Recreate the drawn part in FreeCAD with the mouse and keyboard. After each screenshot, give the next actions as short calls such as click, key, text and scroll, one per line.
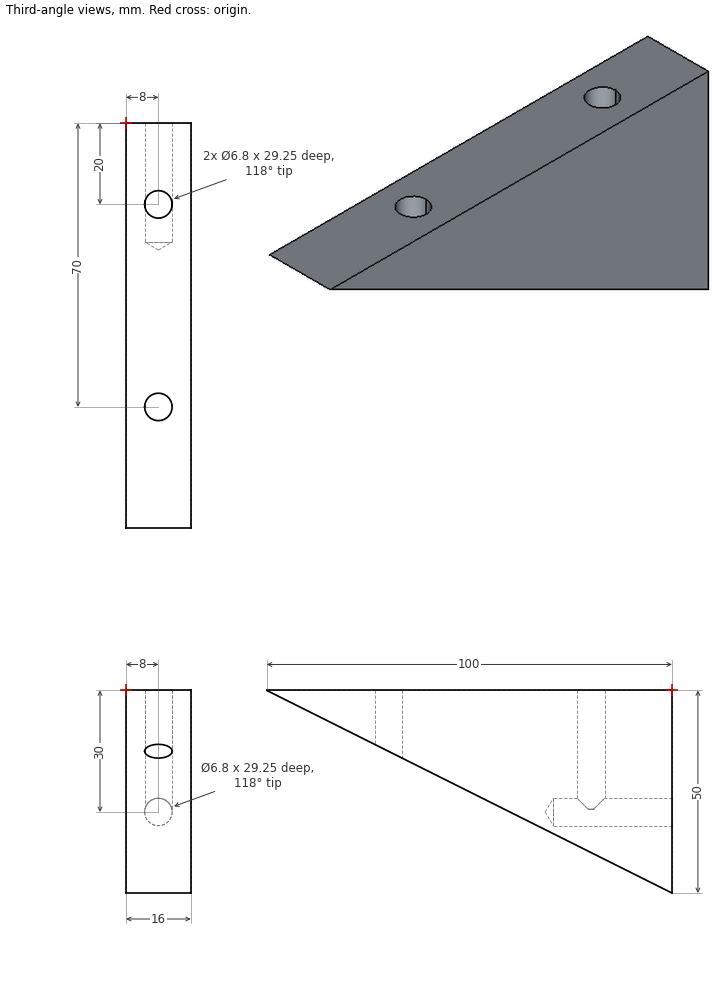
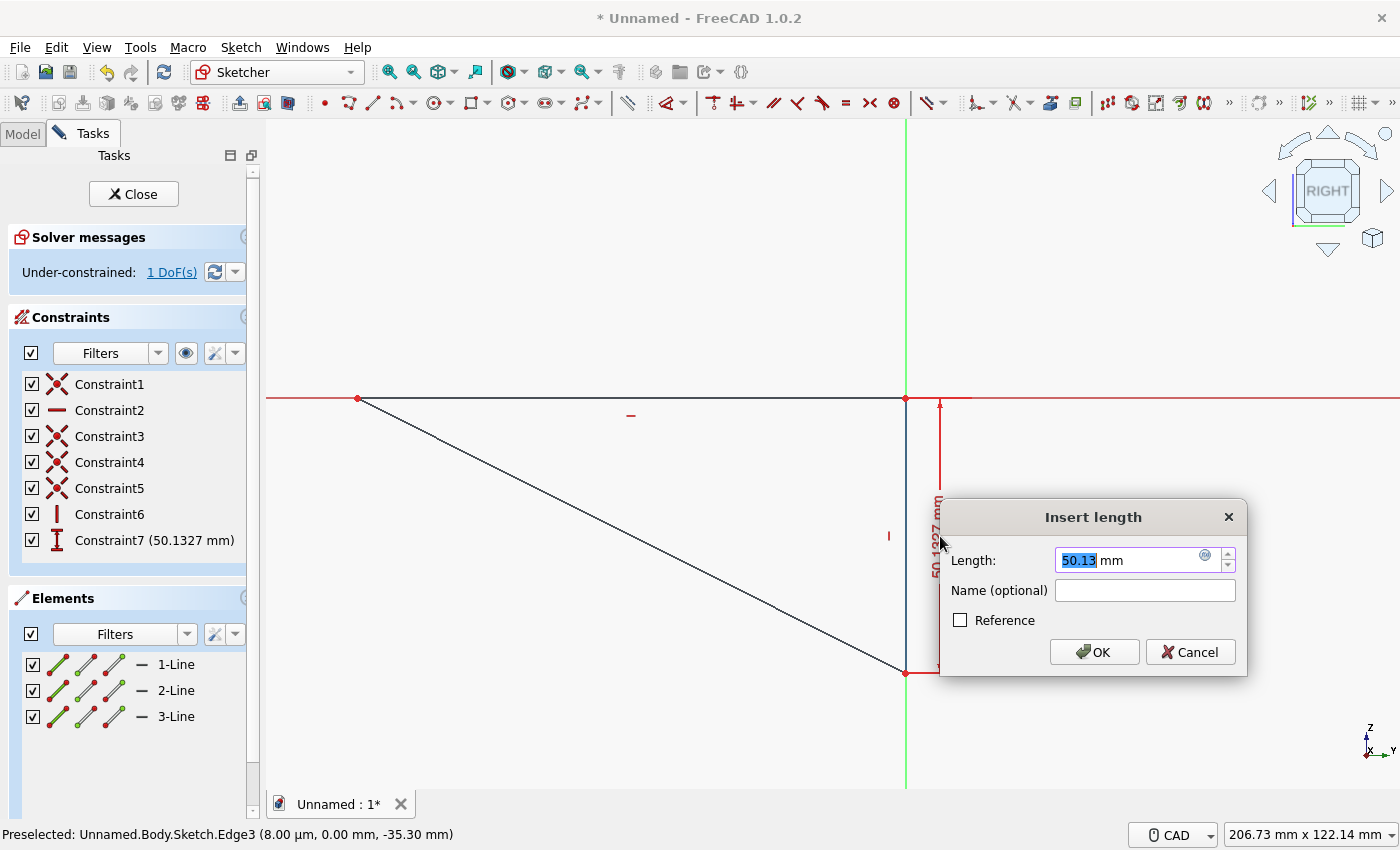
text(50)
key(Return)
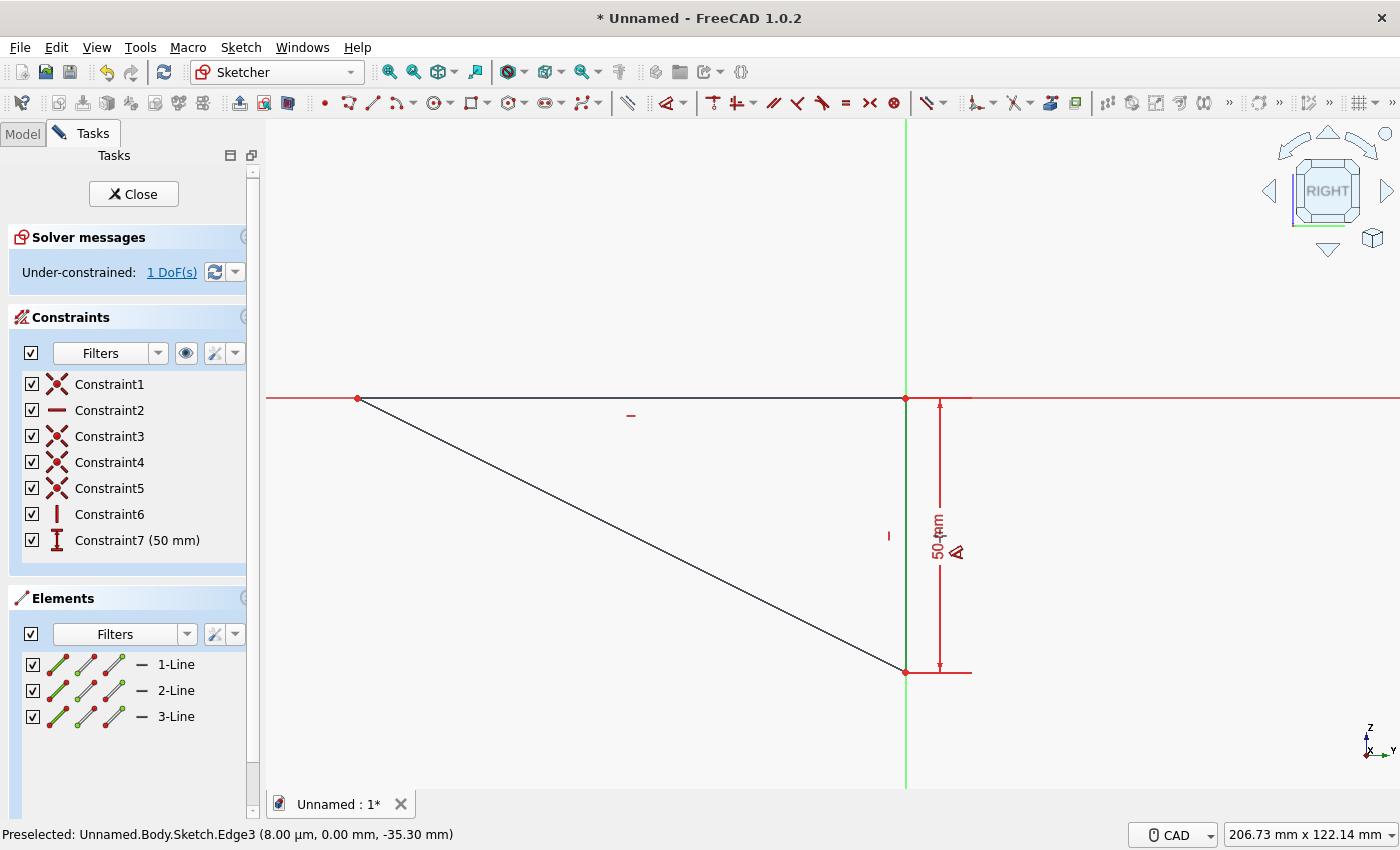
click(741, 398)
click(632, 364)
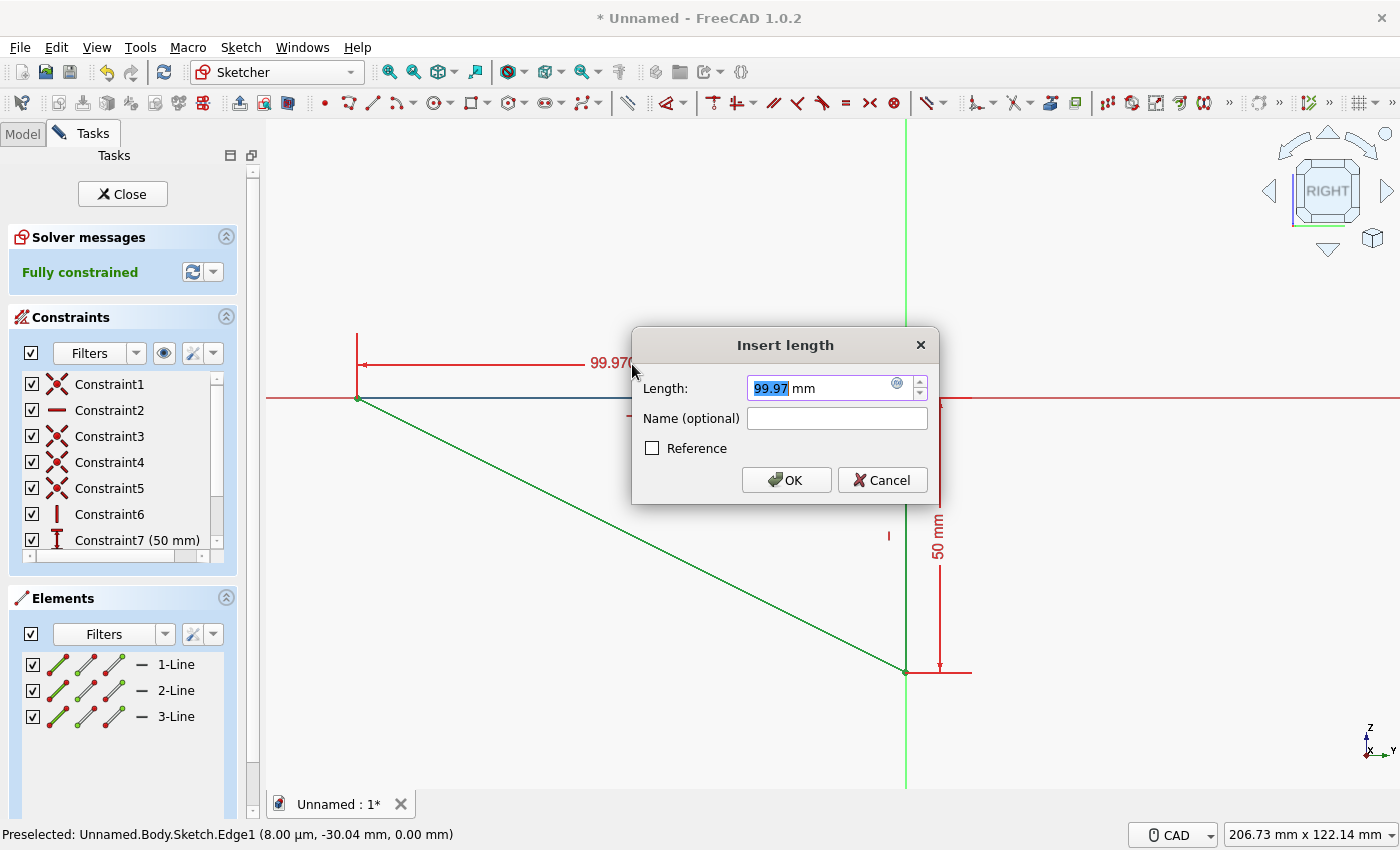
text(100)
key(Return)
key(Escape)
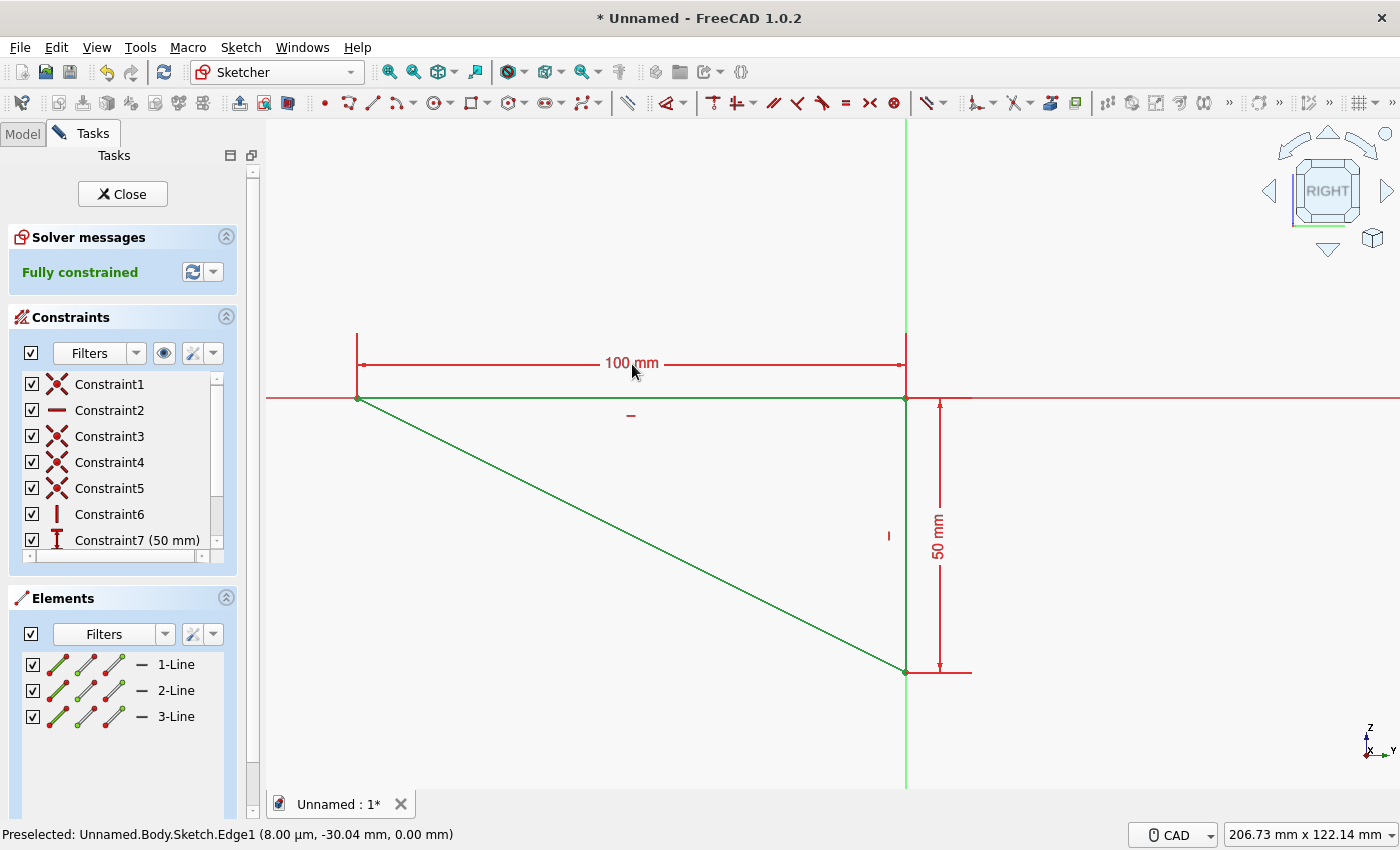
click(123, 194)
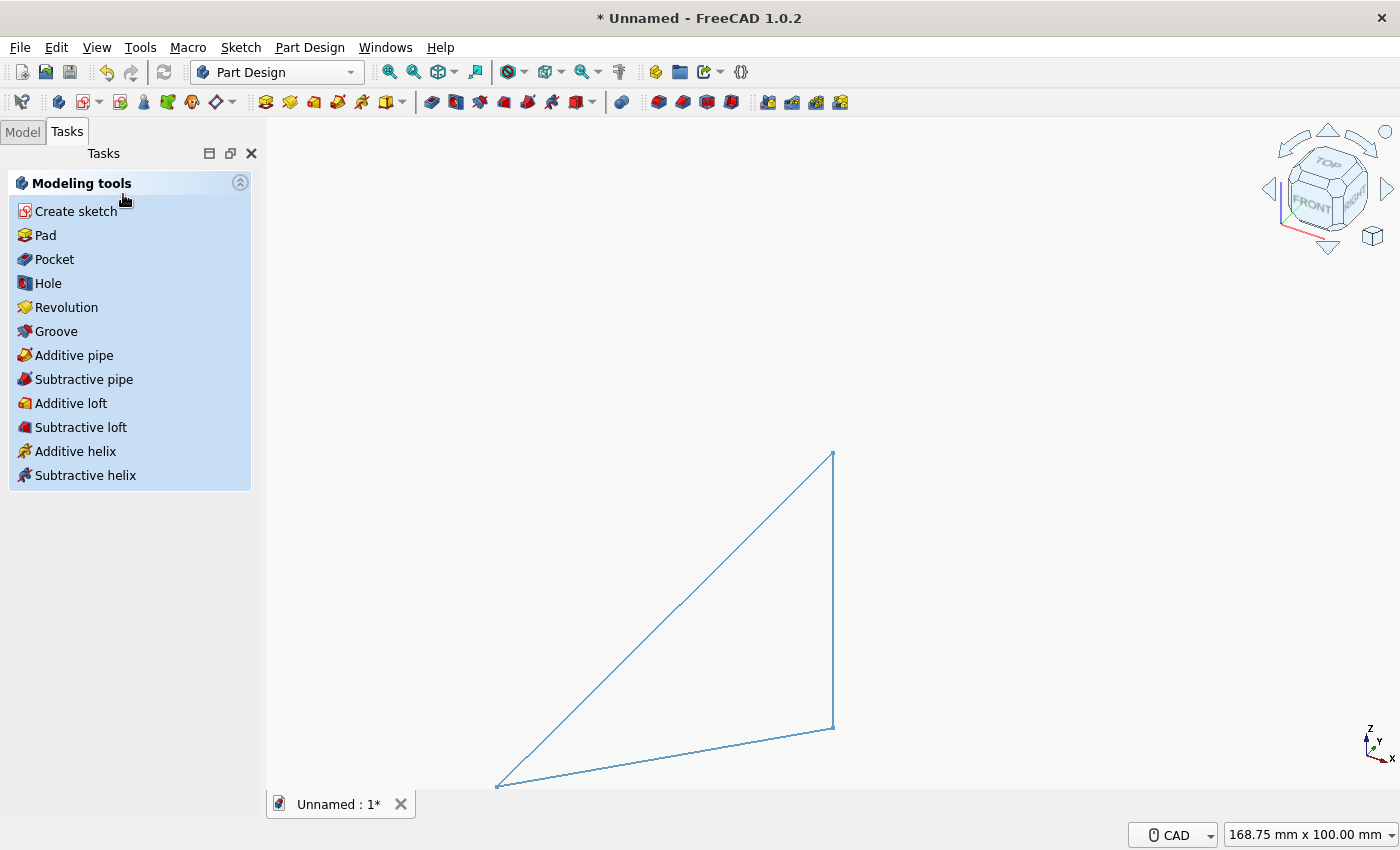
click(266, 102)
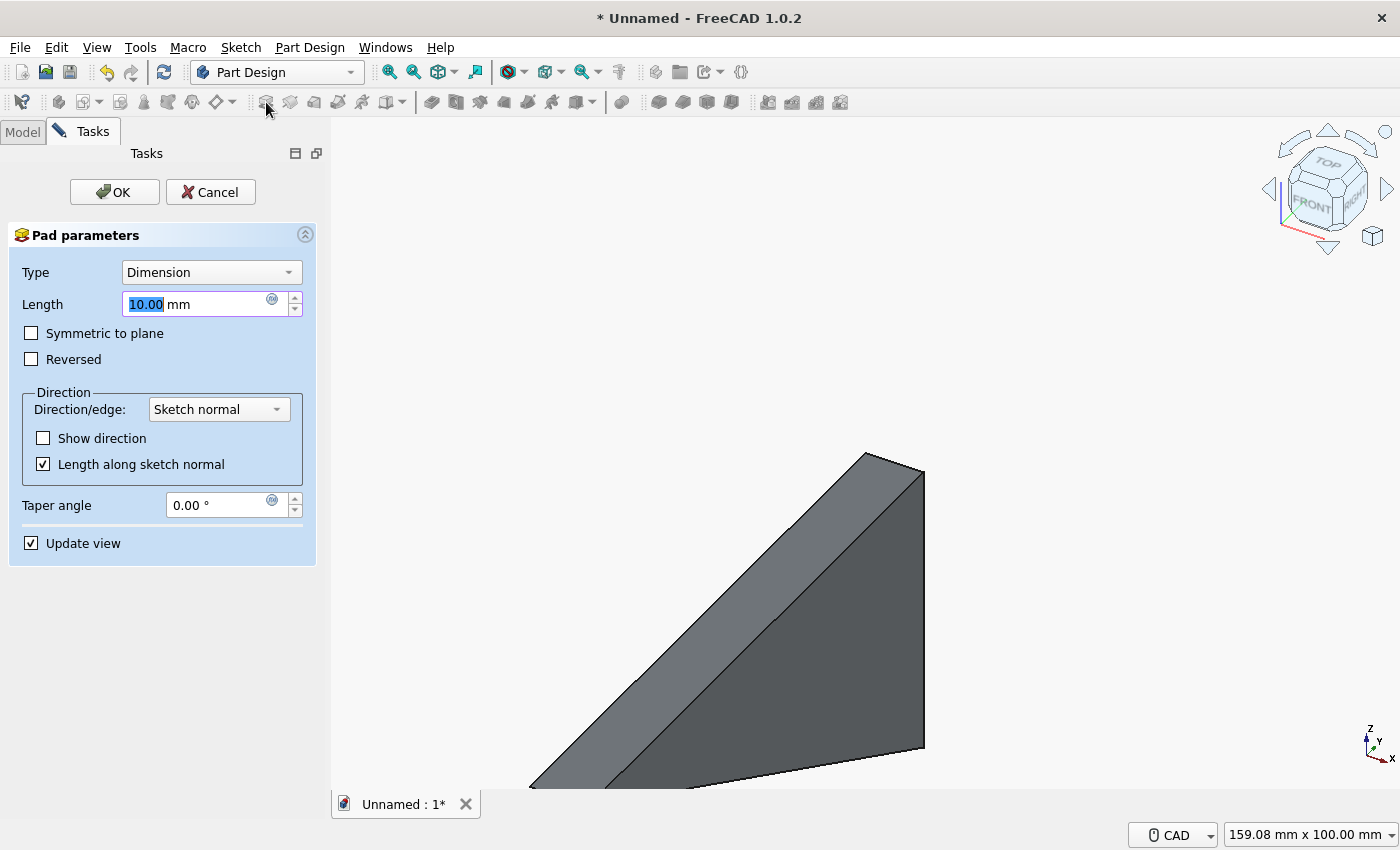
text(16)
key(Tab)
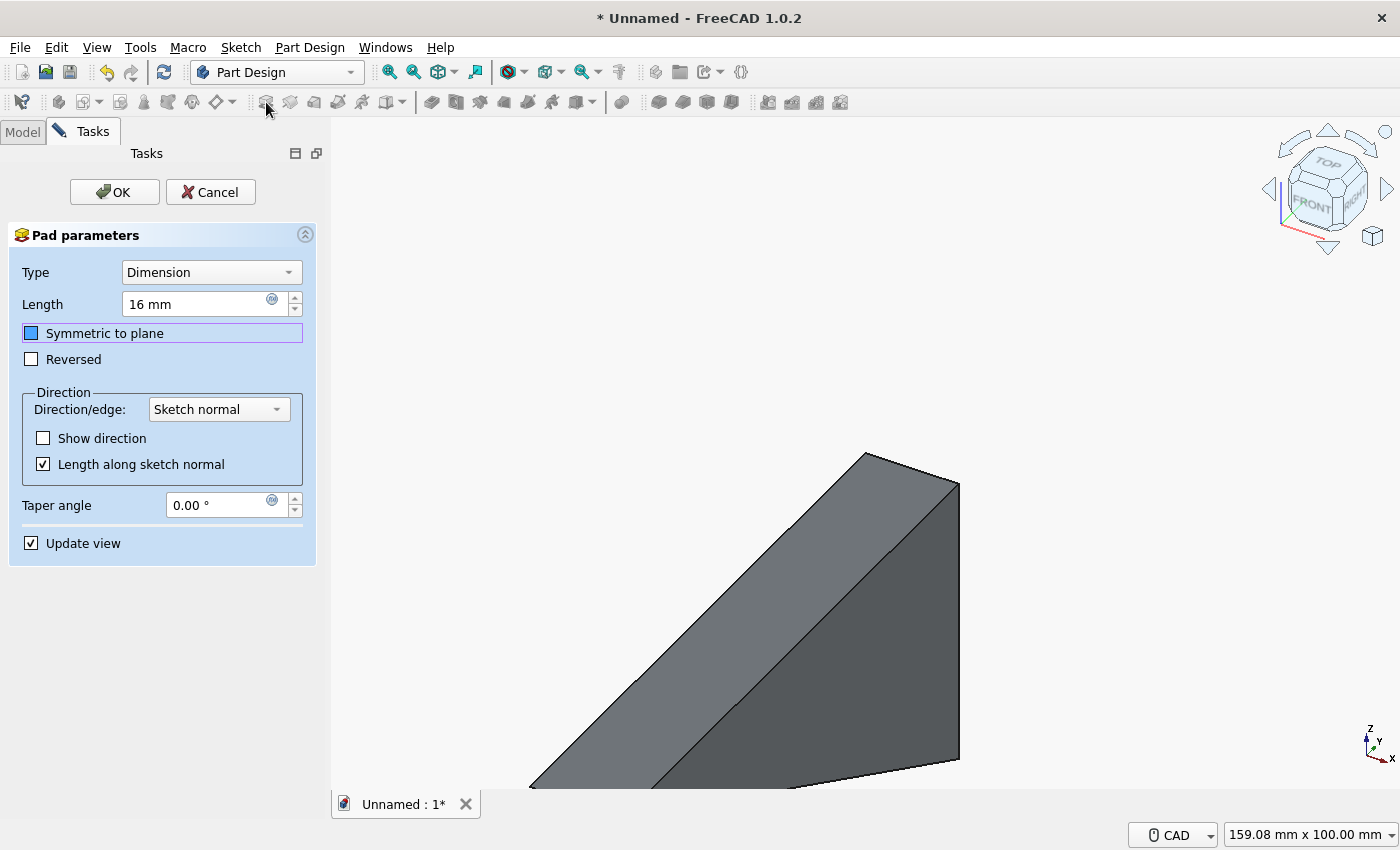
click(115, 192)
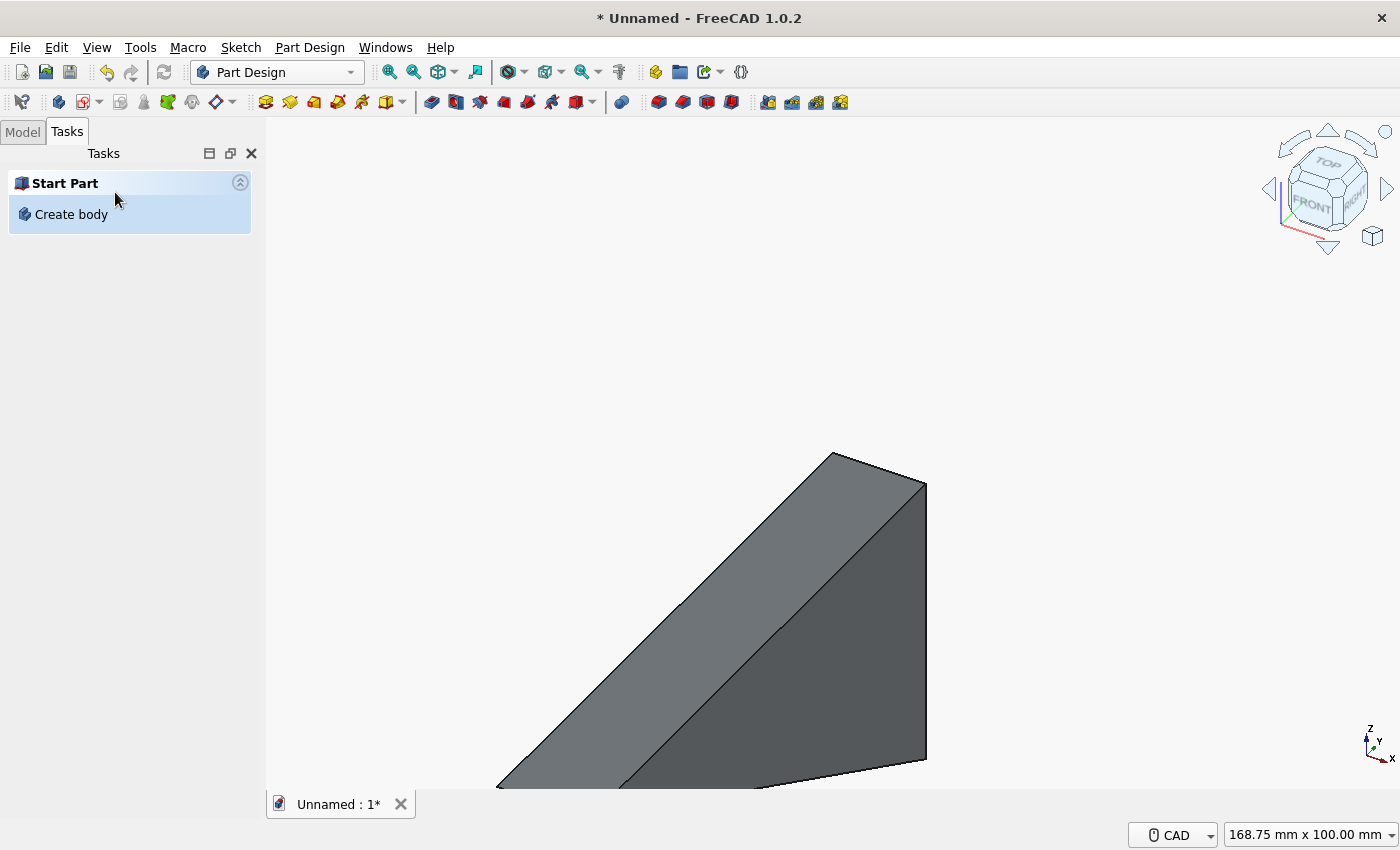
click(390, 72)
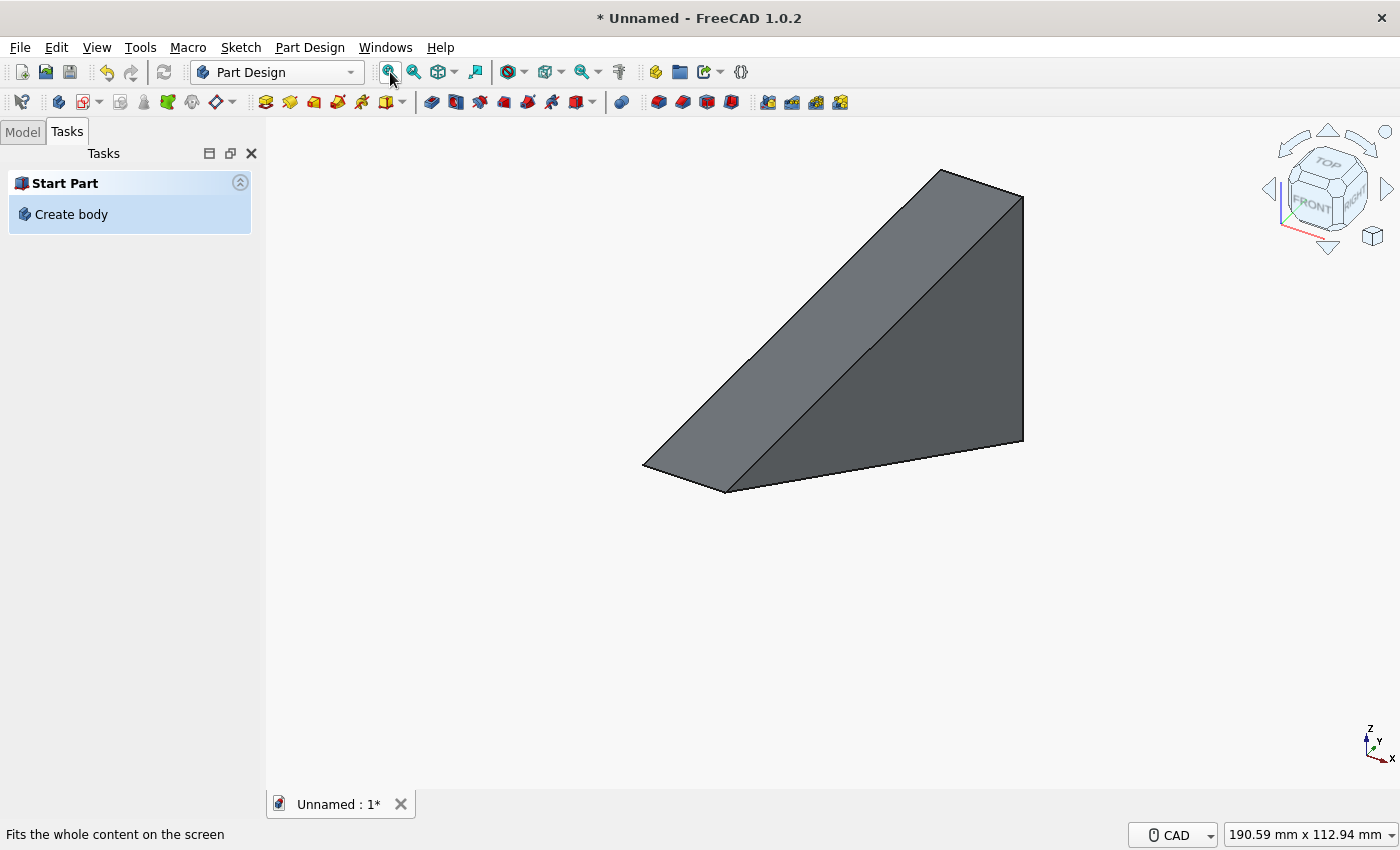
click(84, 102)